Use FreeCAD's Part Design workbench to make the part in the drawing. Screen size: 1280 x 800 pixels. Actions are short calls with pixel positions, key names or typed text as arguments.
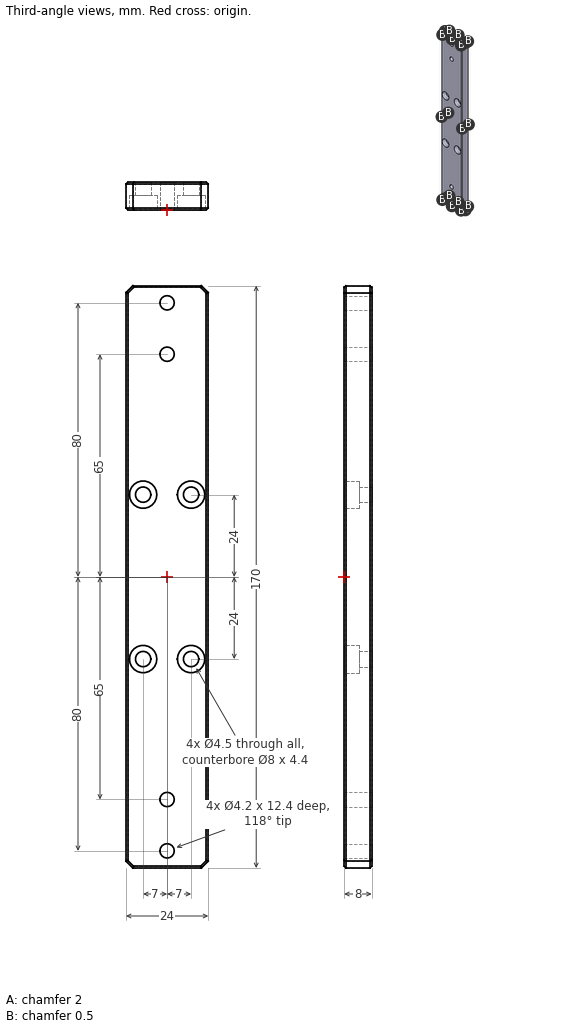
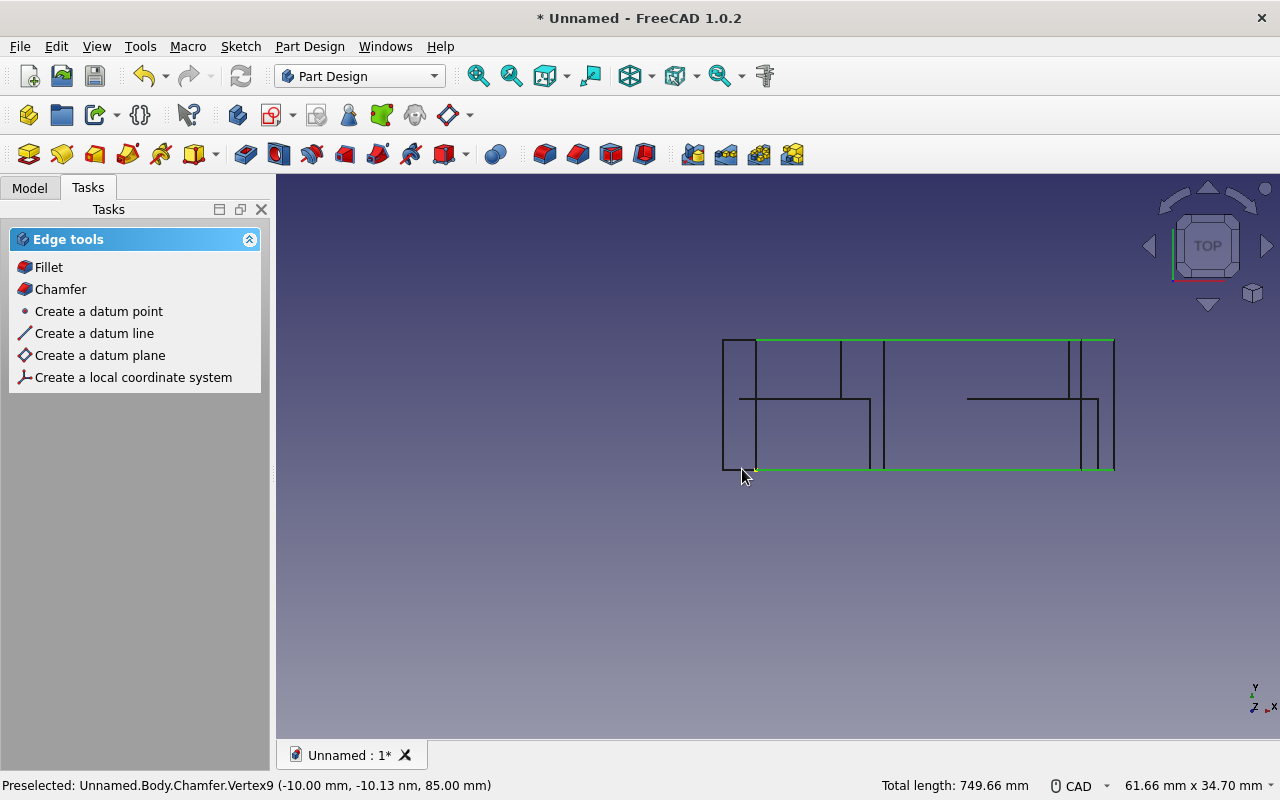
click(739, 469, ctrl)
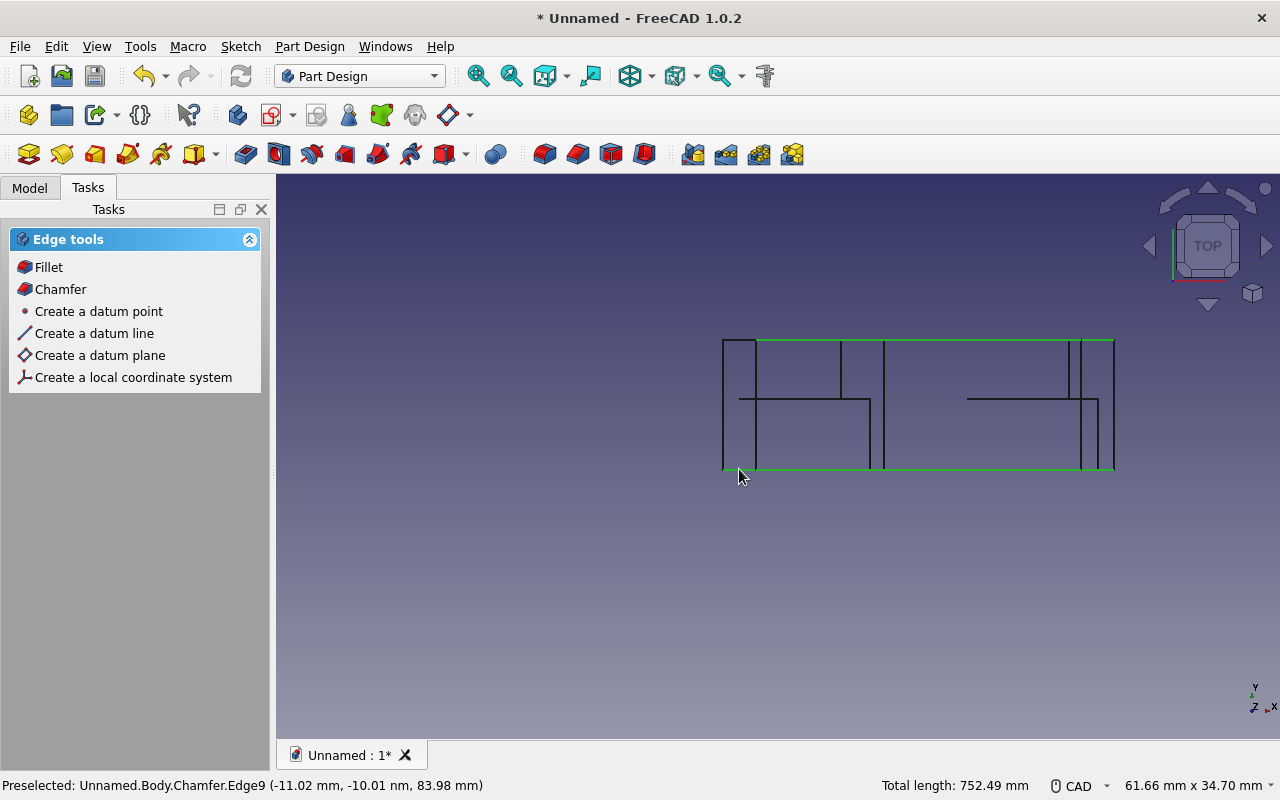
click(739, 339, ctrl)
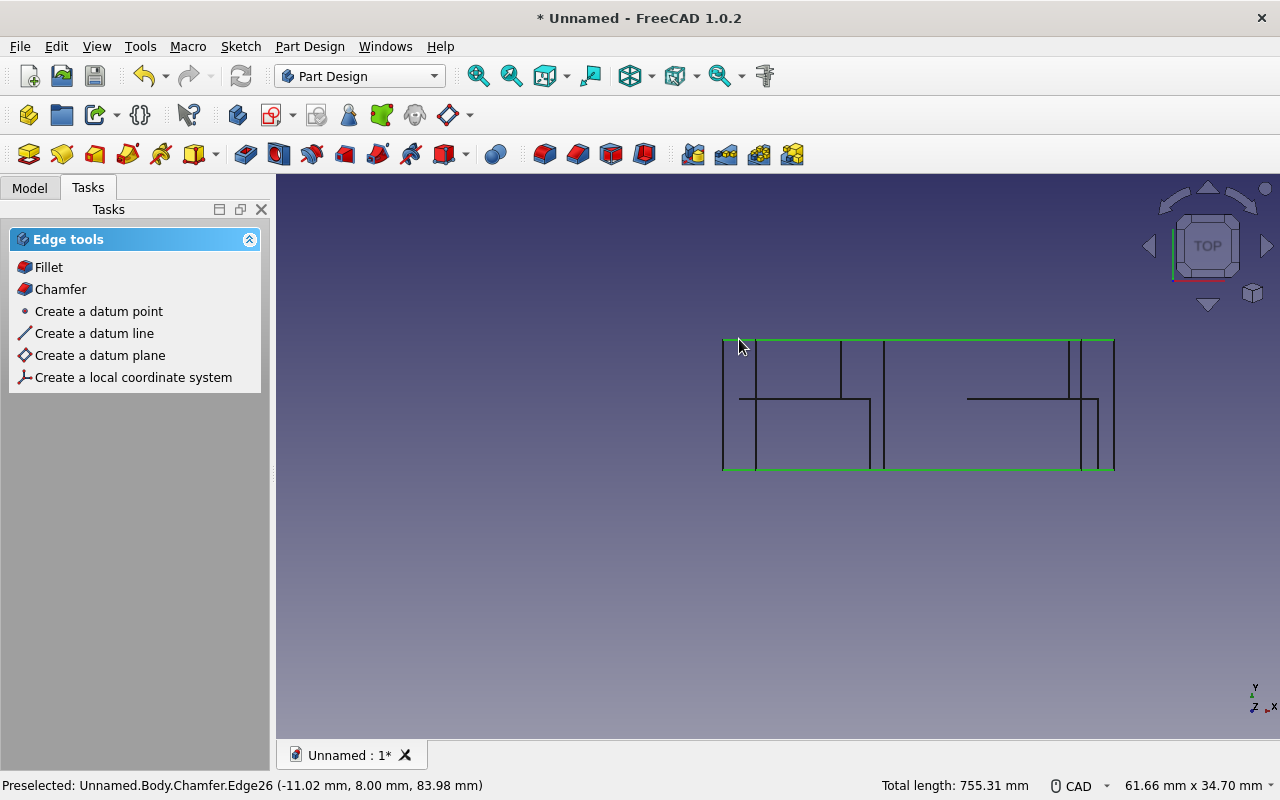
click(479, 76)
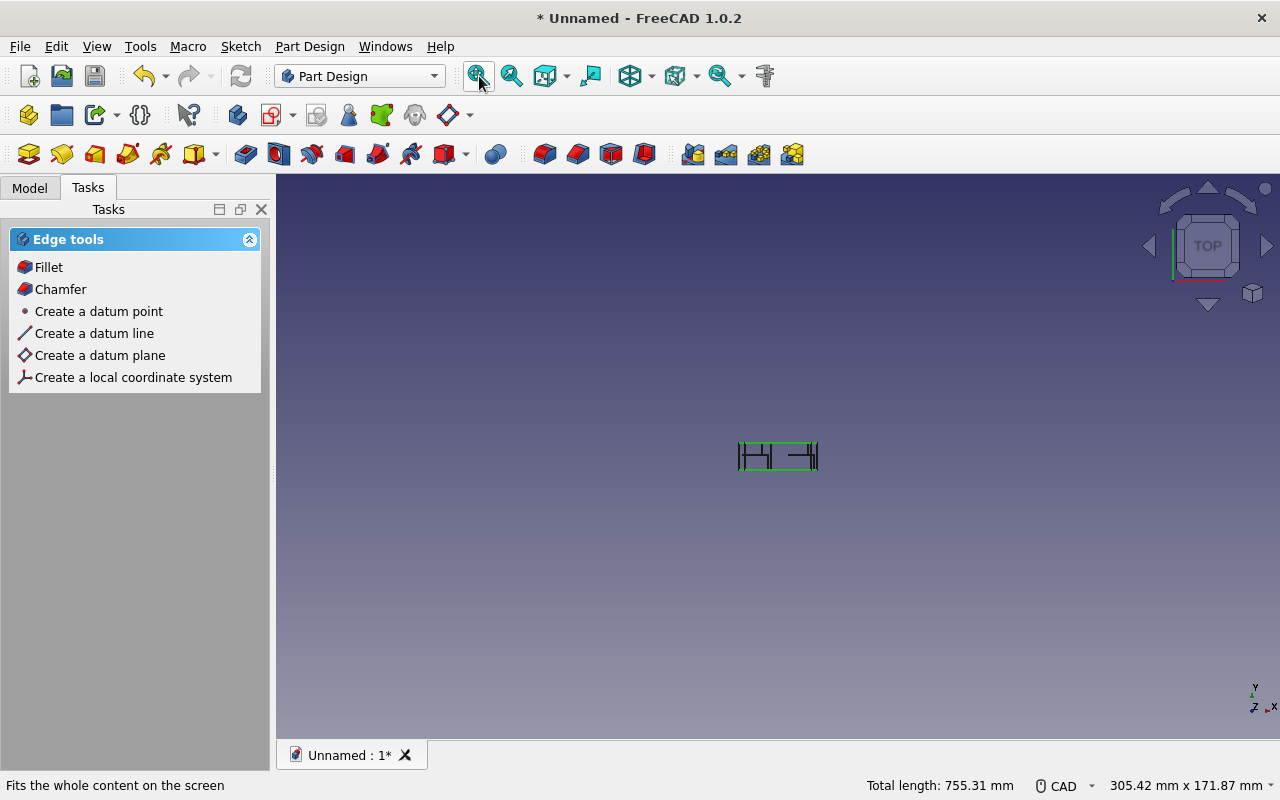
key(1)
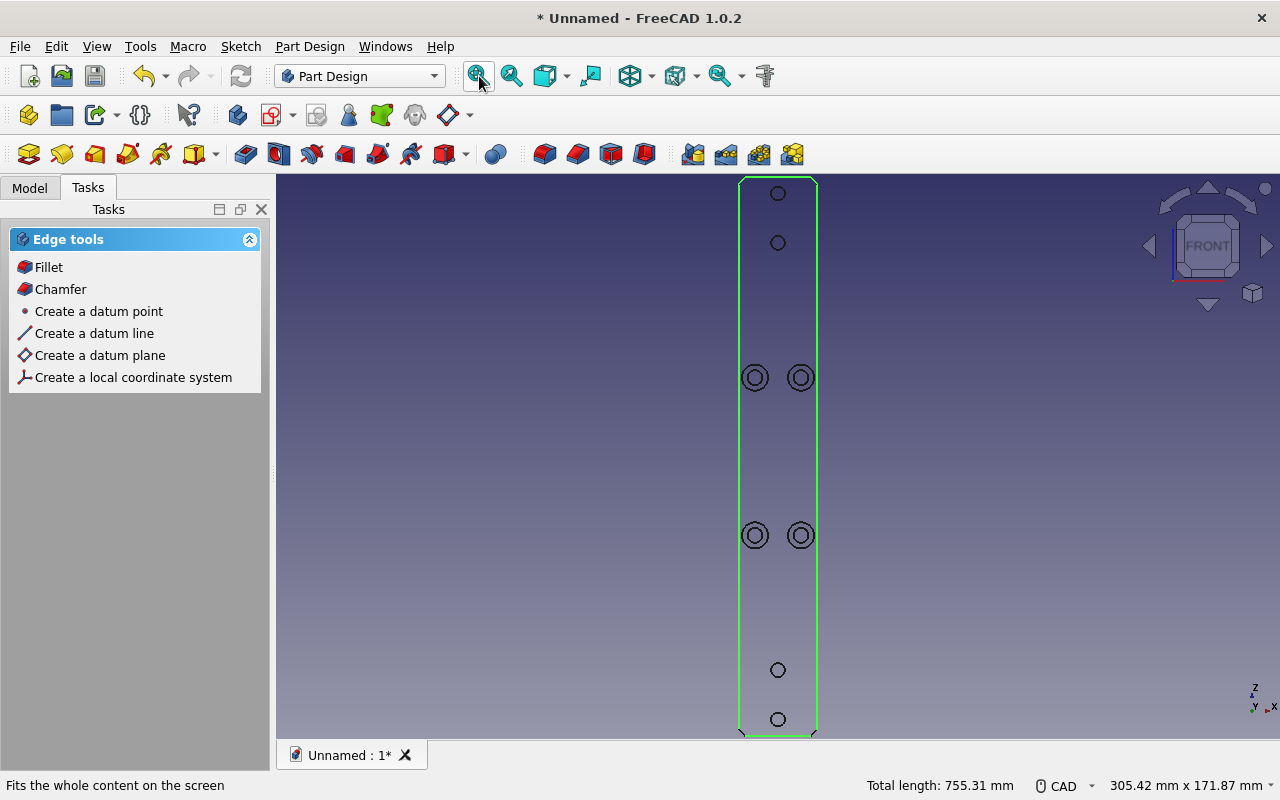
key(3)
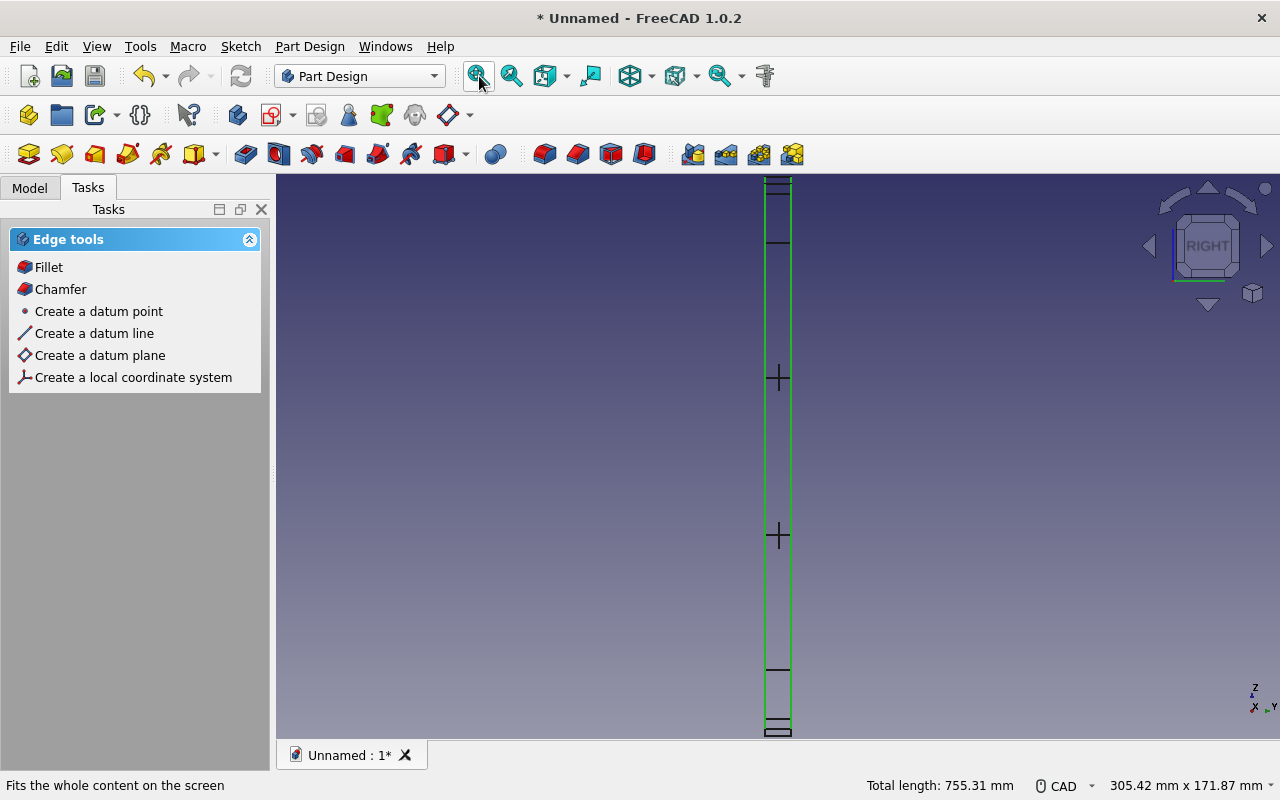
key(5)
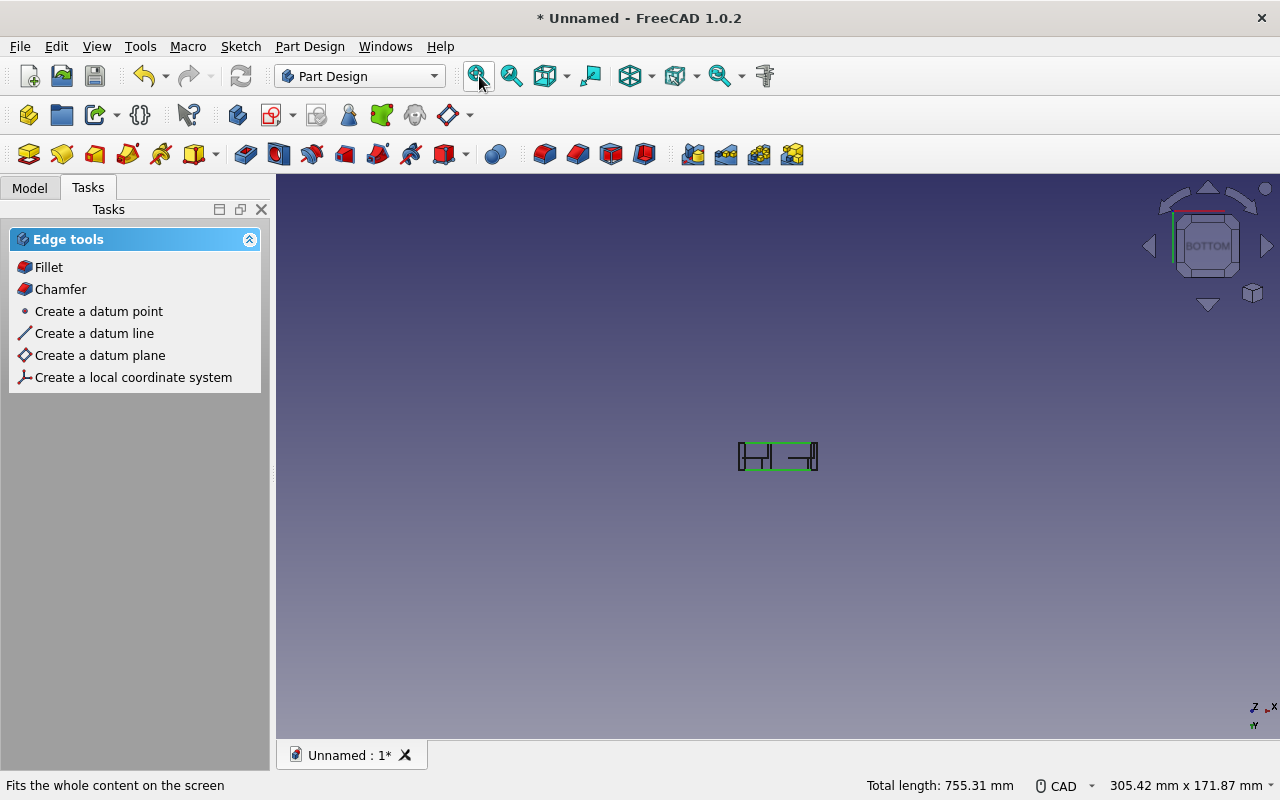
key(v)
key(f)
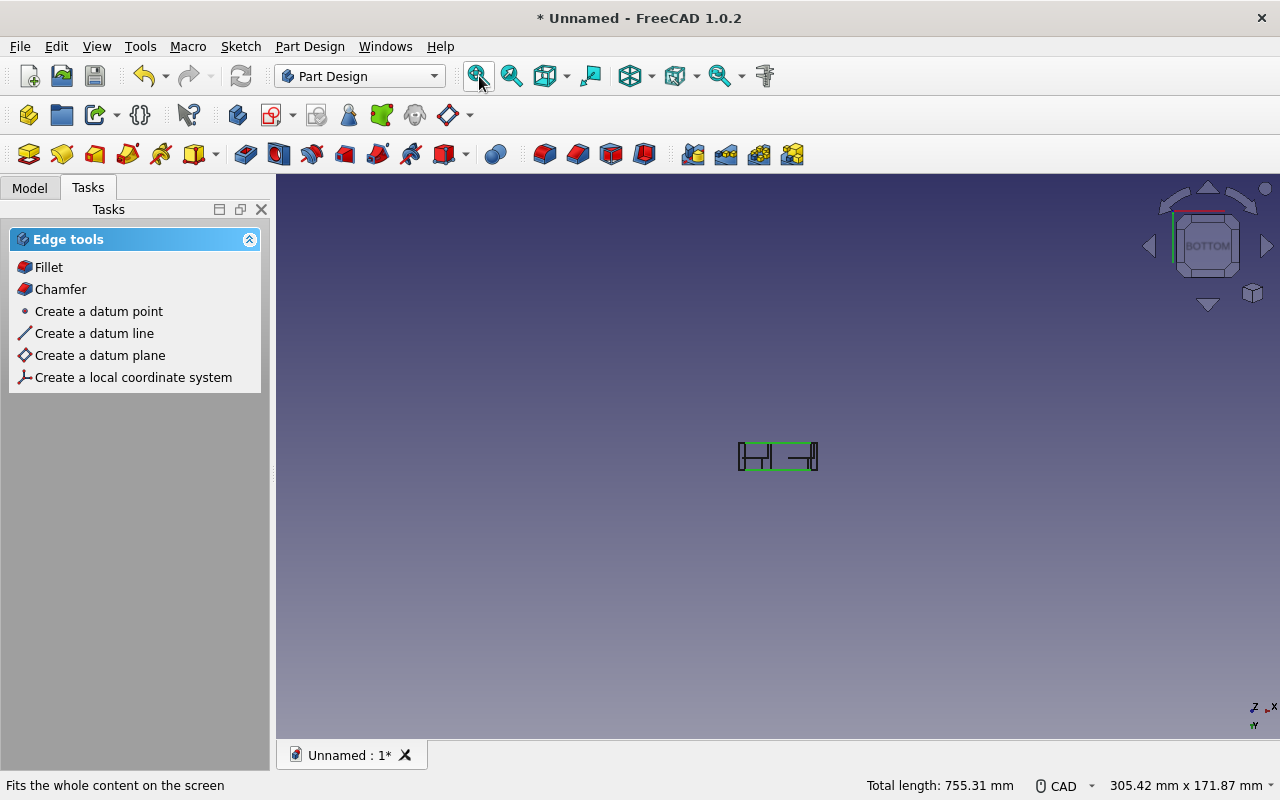
scroll(814, 442, up, 8)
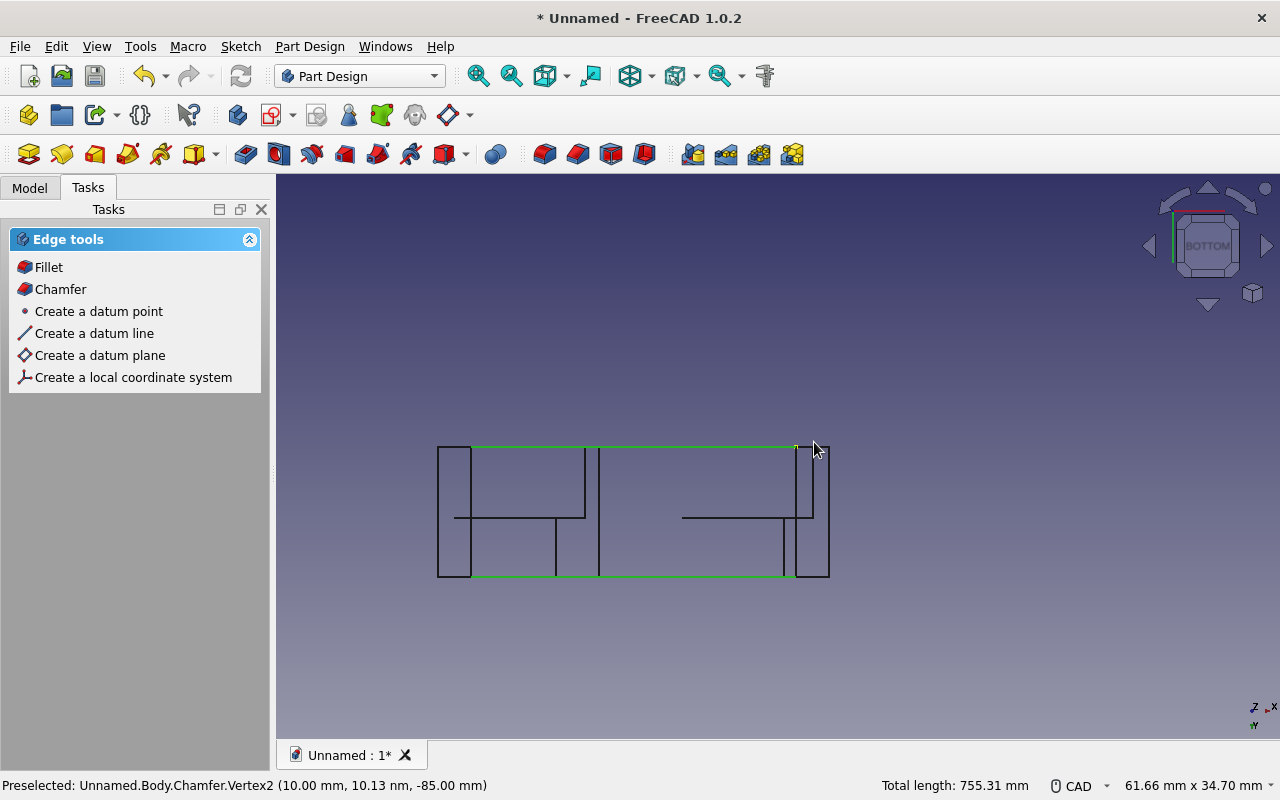
click(813, 446, ctrl)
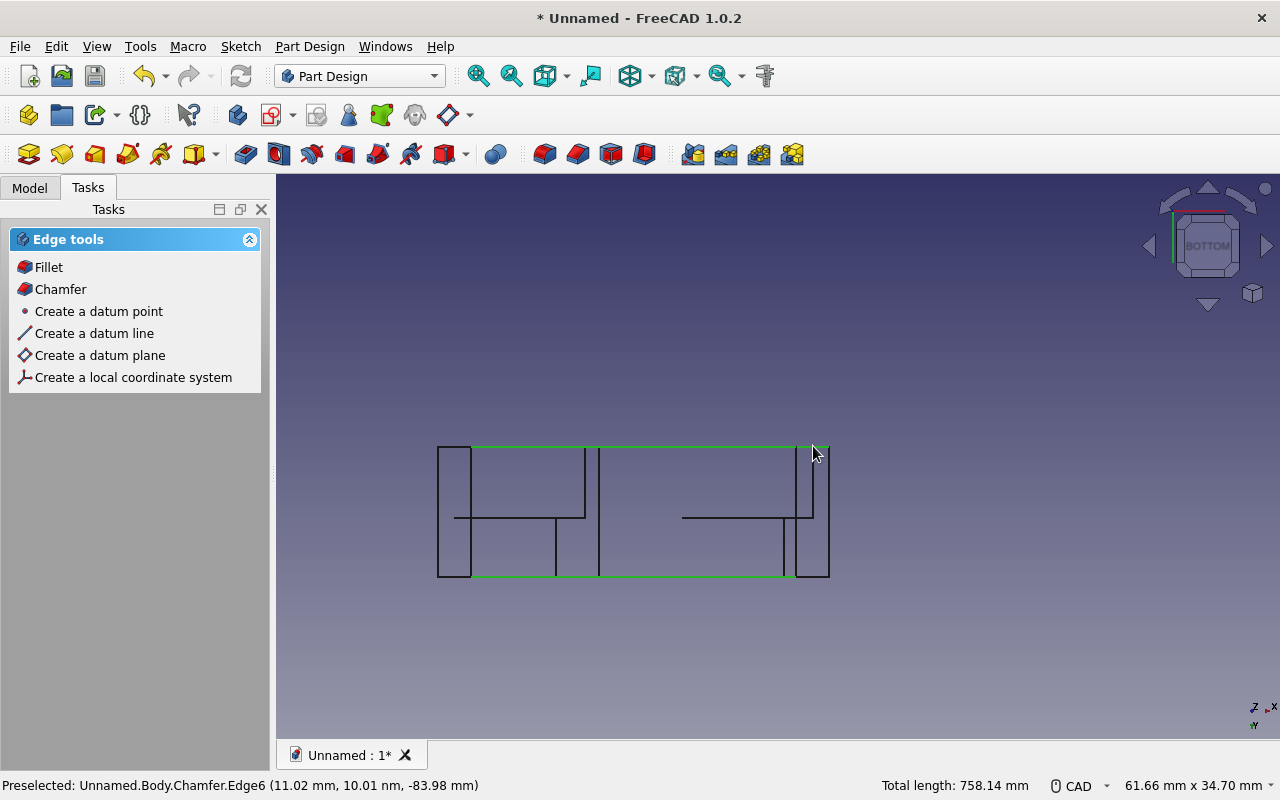
click(454, 446, ctrl)